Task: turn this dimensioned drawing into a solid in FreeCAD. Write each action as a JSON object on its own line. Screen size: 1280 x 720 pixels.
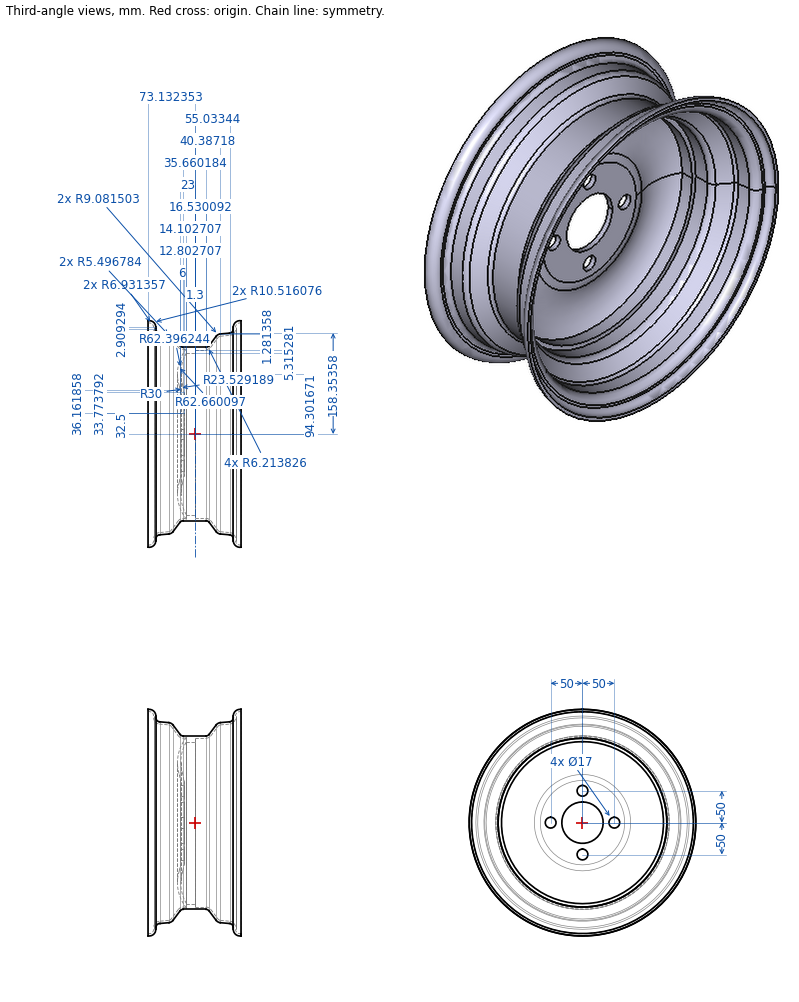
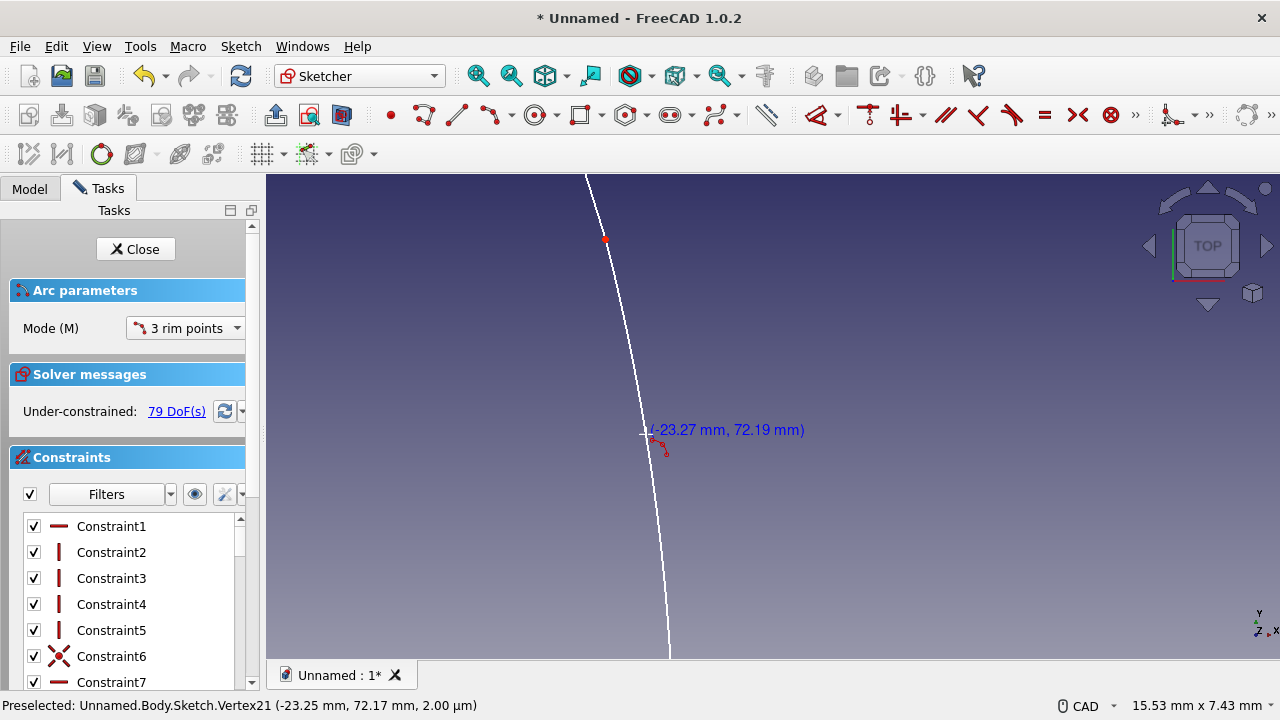
{"action": "scroll", "coordinate": [663, 447], "scroll_direction": "down", "scroll_amount": 18}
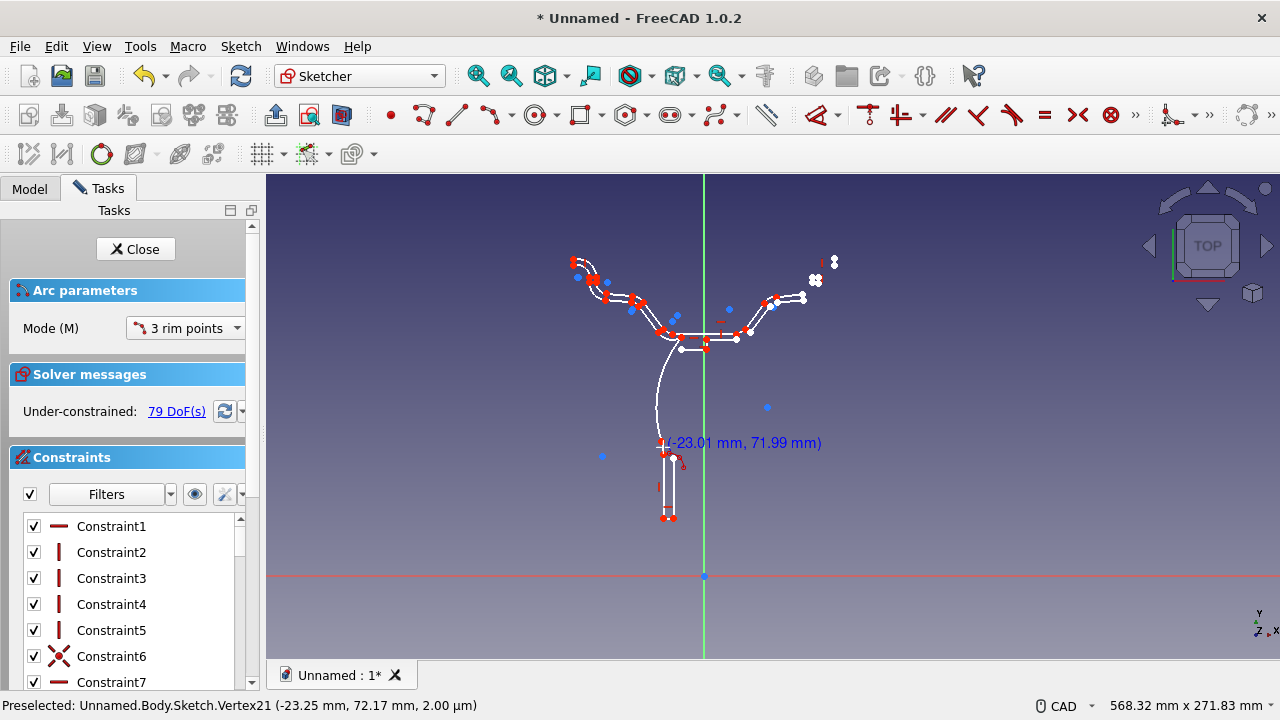
{"action": "scroll", "coordinate": [674, 458], "scroll_direction": "up", "scroll_amount": 2}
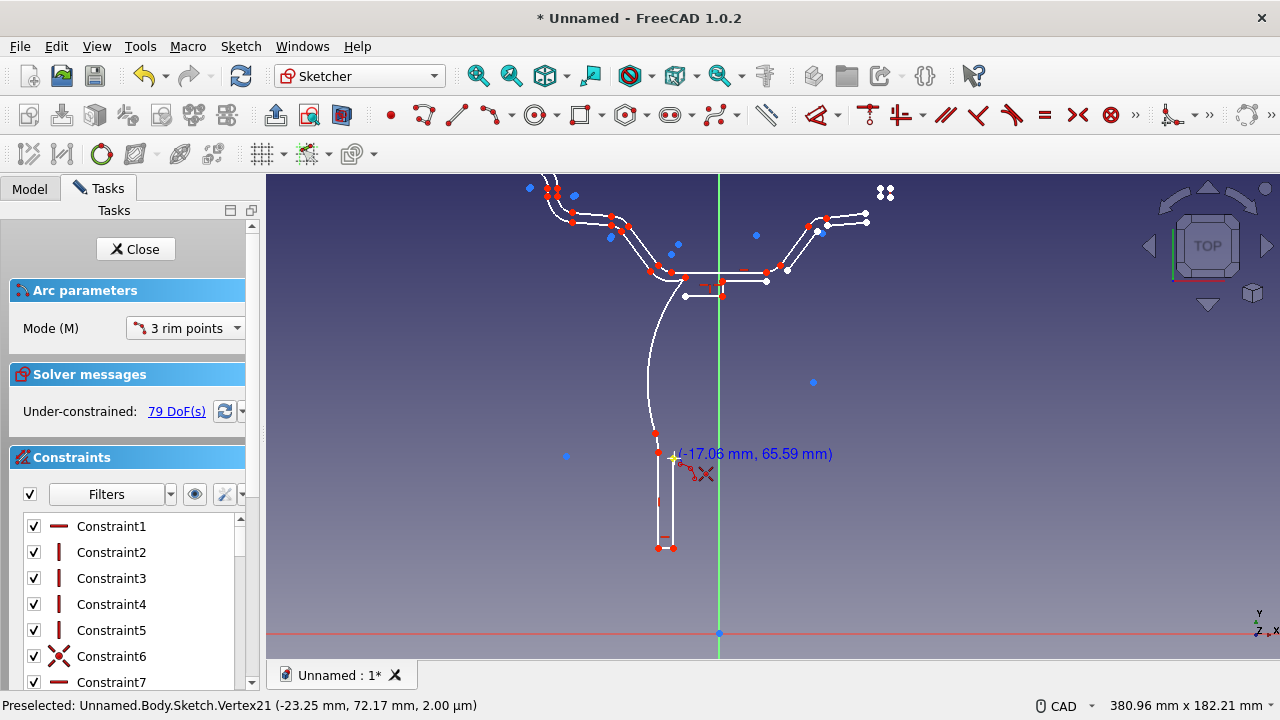
{"action": "left_click", "coordinate": [673, 458]}
{"action": "left_click", "coordinate": [670, 432]}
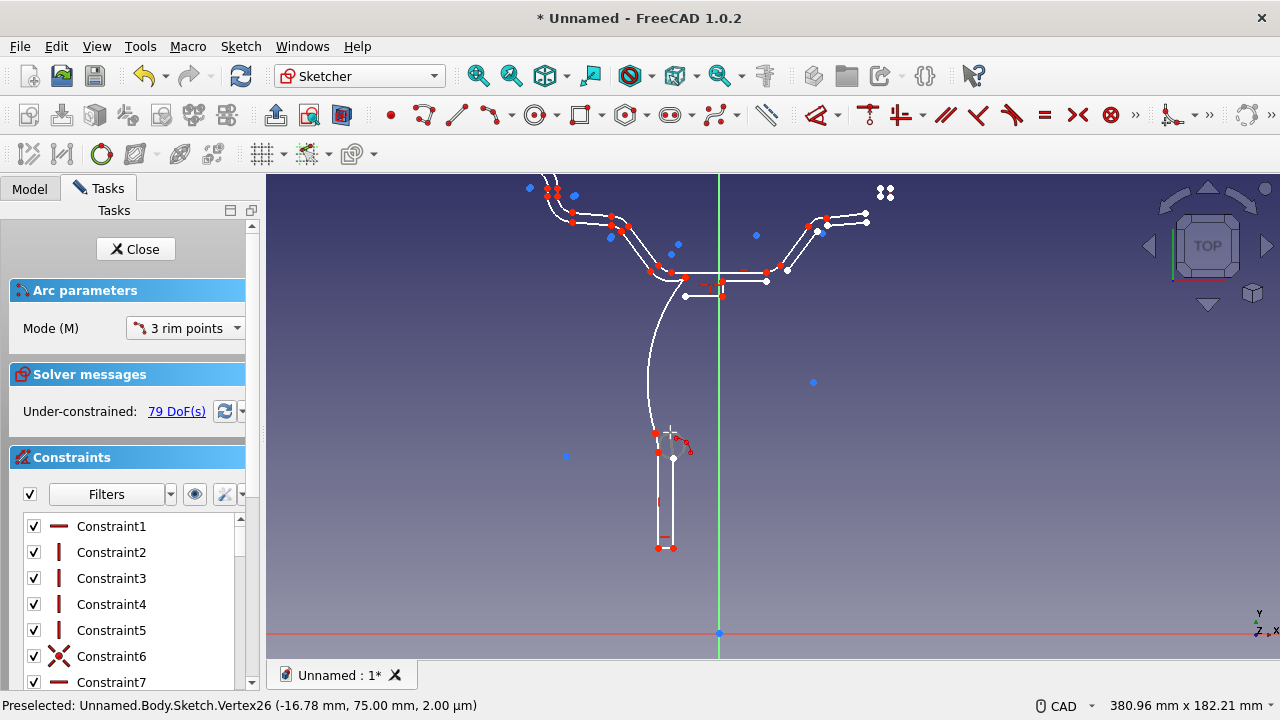
{"action": "scroll", "coordinate": [673, 445], "scroll_direction": "up", "scroll_amount": 14}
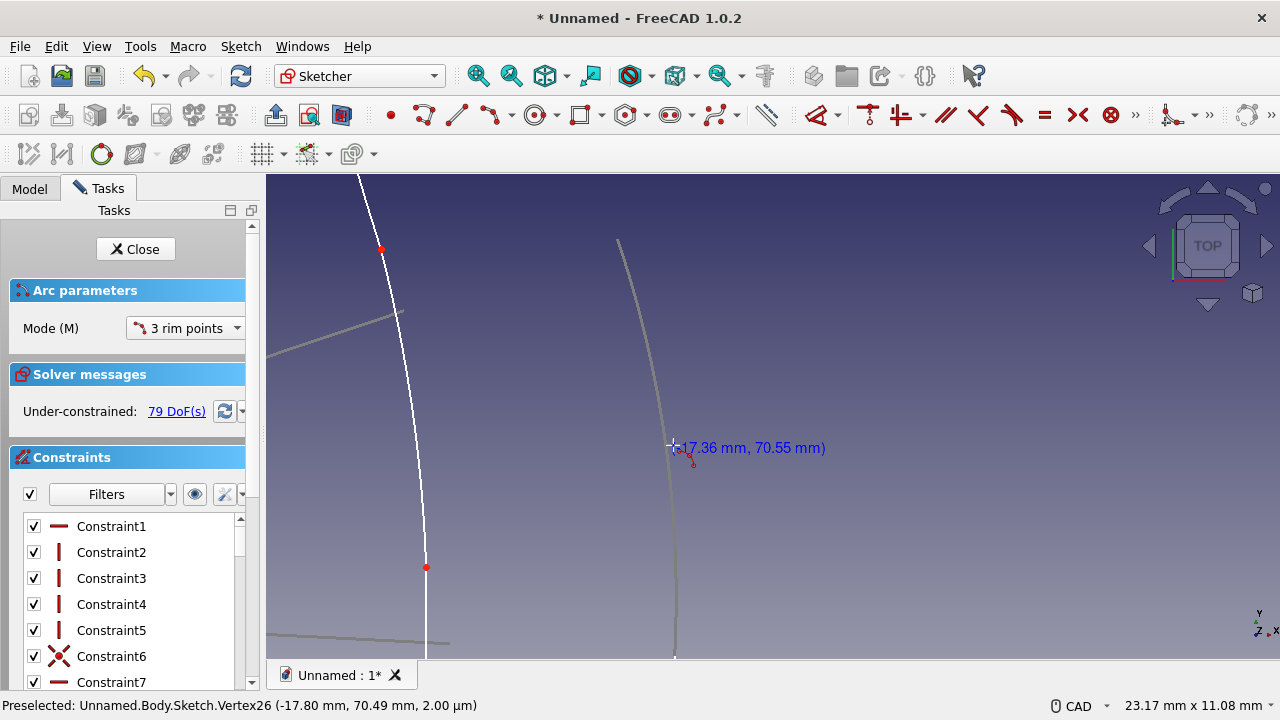
{"action": "left_click", "coordinate": [666, 432]}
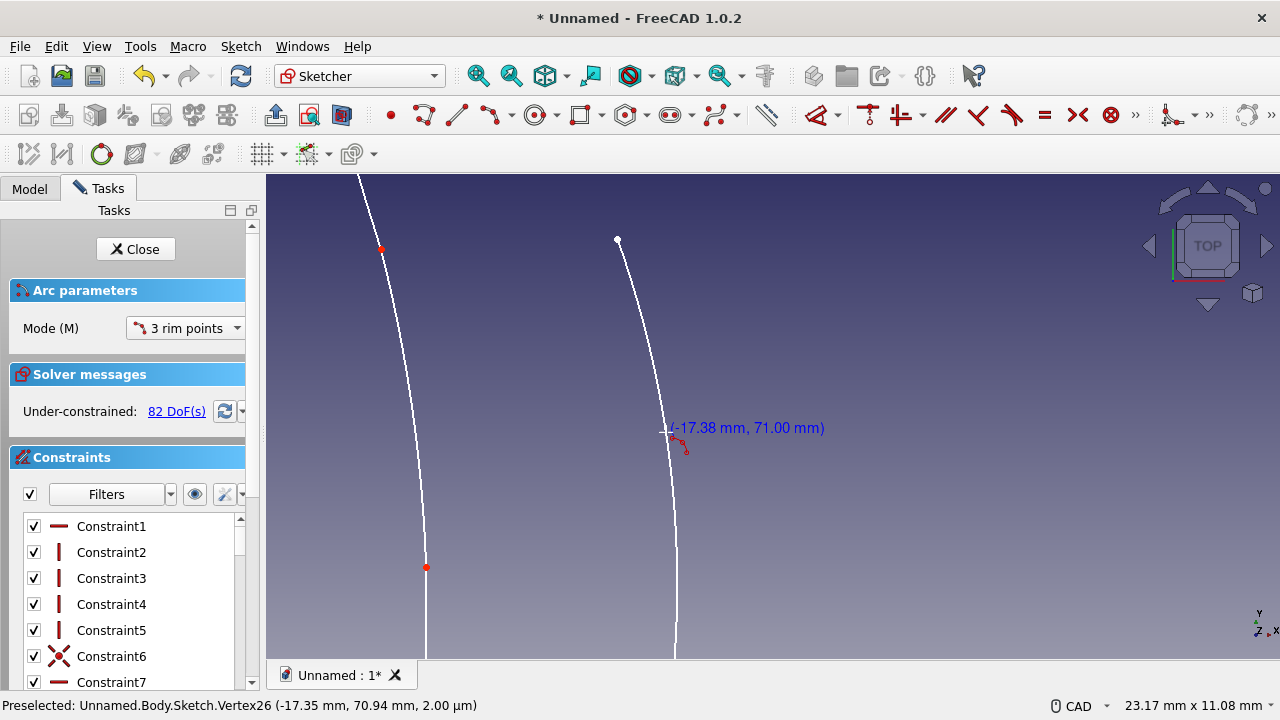
{"action": "scroll", "coordinate": [674, 449], "scroll_direction": "down", "scroll_amount": 16}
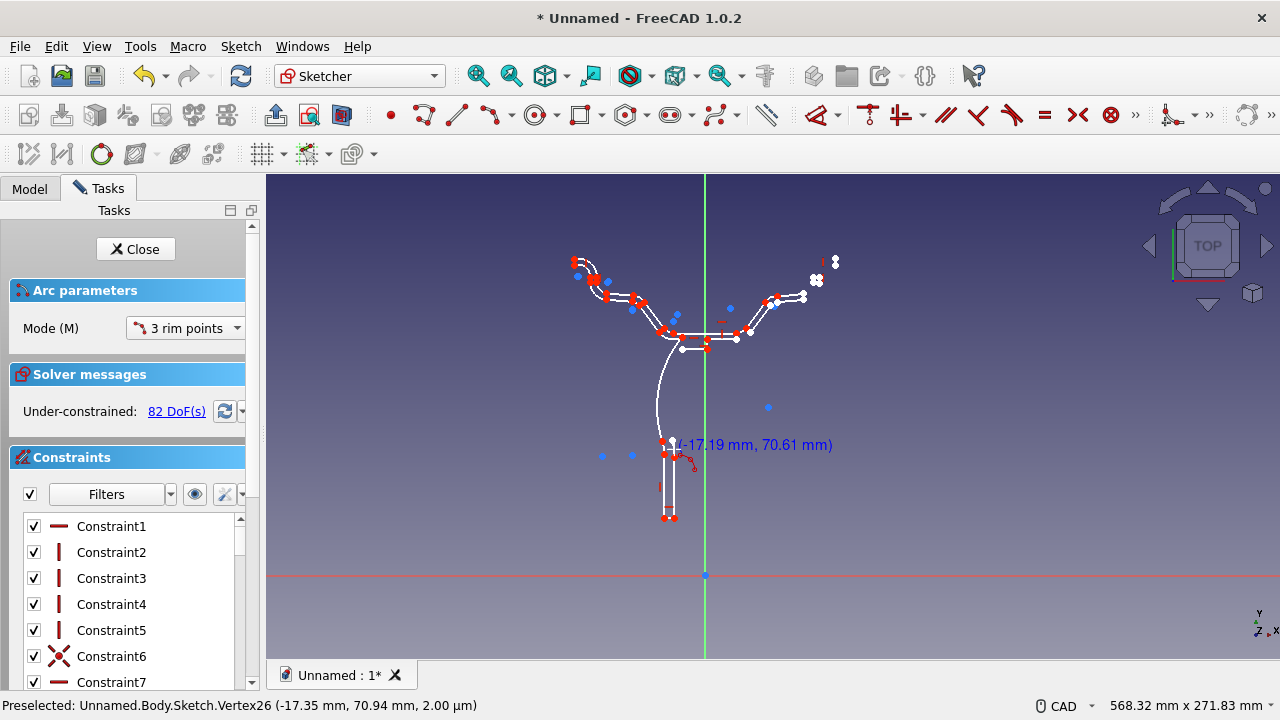
{"action": "scroll", "coordinate": [672, 441], "scroll_direction": "up", "scroll_amount": 3}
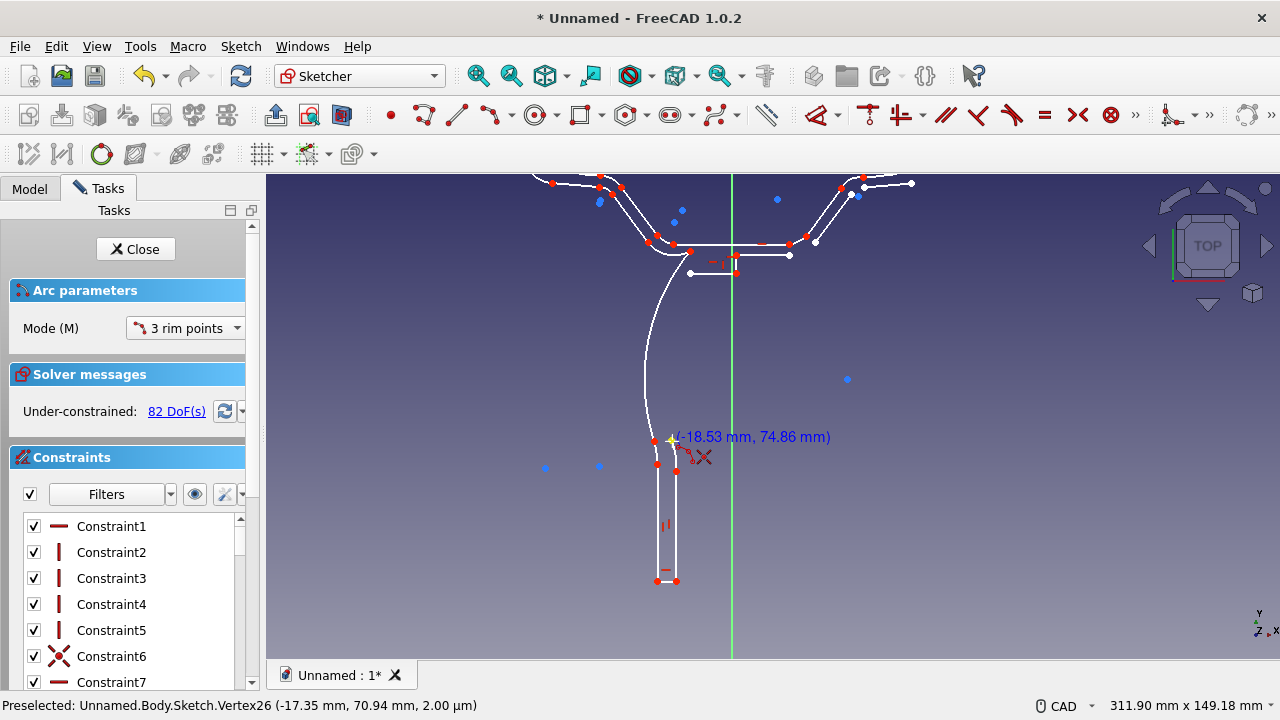
{"action": "left_click", "coordinate": [672, 441]}
{"action": "left_click", "coordinate": [691, 274]}
{"action": "left_click", "coordinate": [662, 371]}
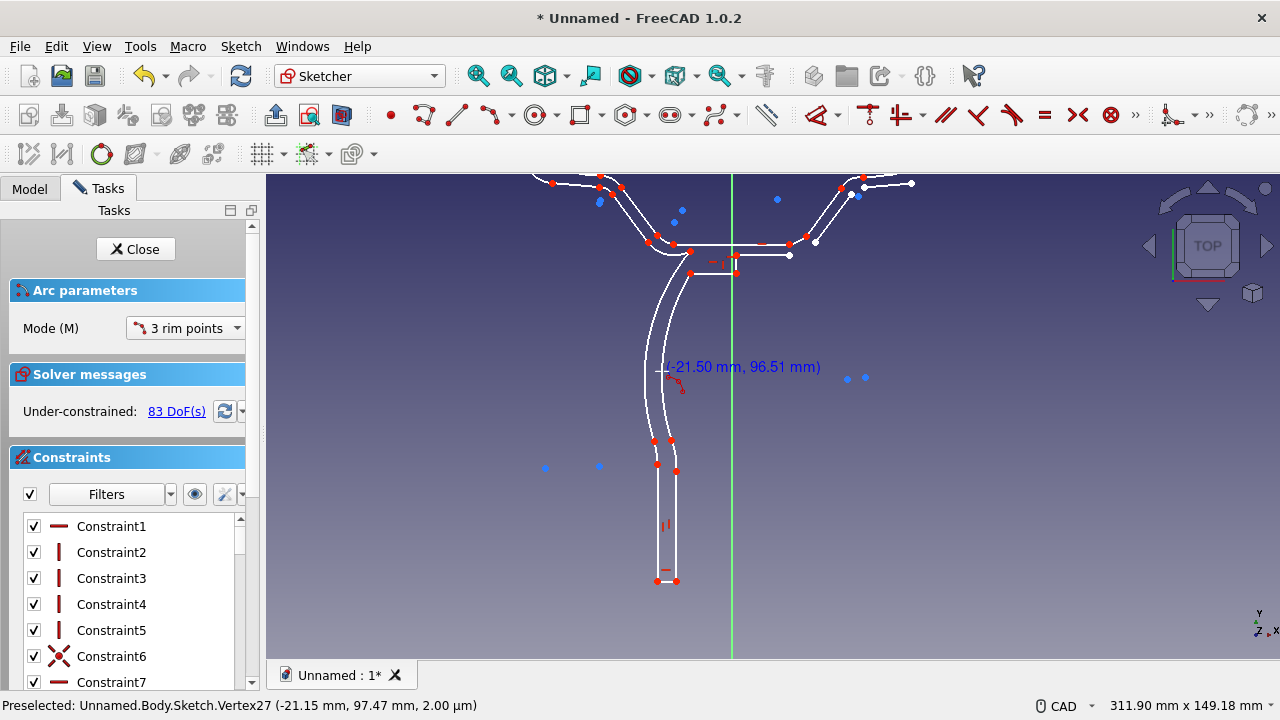
{"action": "scroll", "coordinate": [790, 255], "scroll_direction": "up", "scroll_amount": 2}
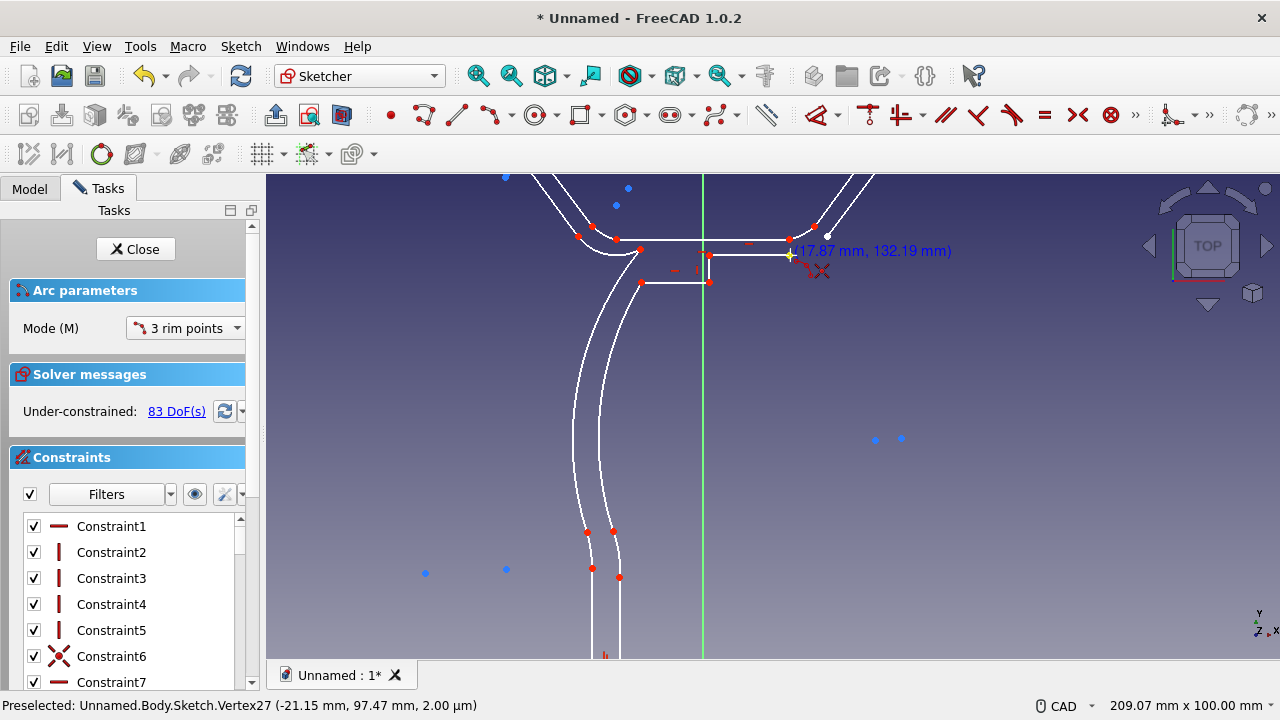
{"action": "left_click", "coordinate": [789, 255]}
{"action": "left_click", "coordinate": [827, 236]}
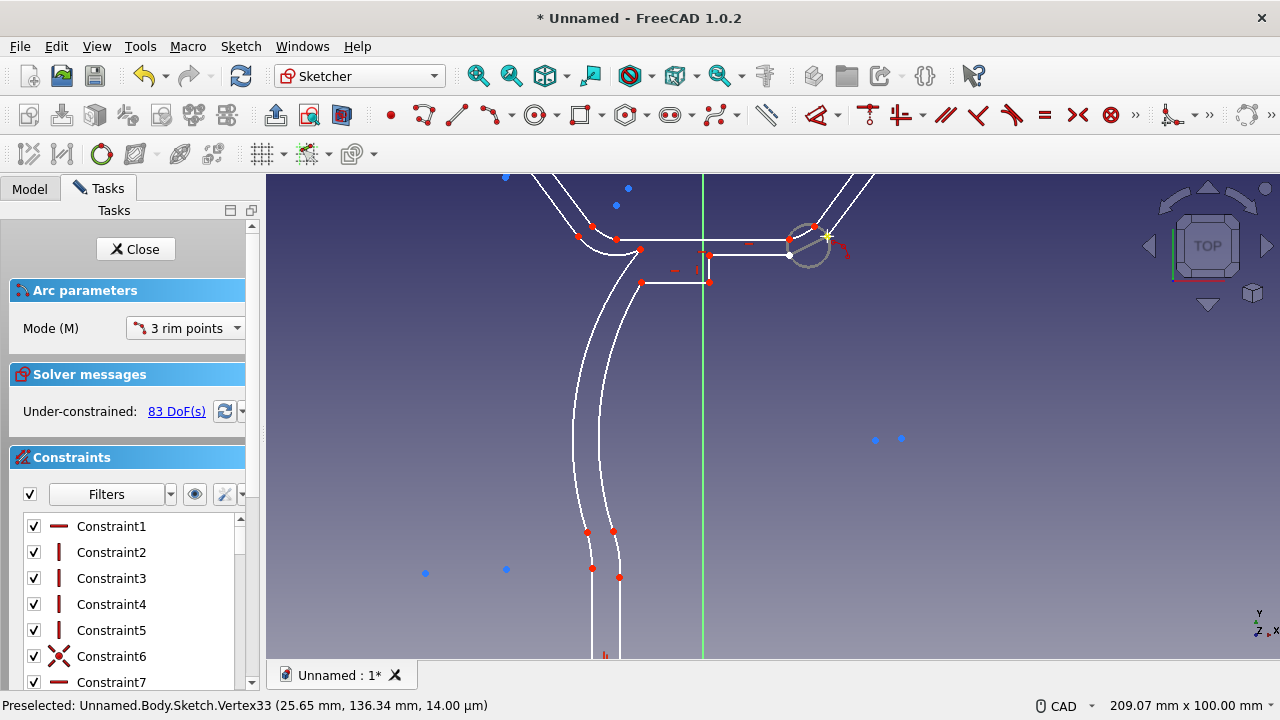
{"action": "scroll", "coordinate": [811, 250], "scroll_direction": "up", "scroll_amount": 6}